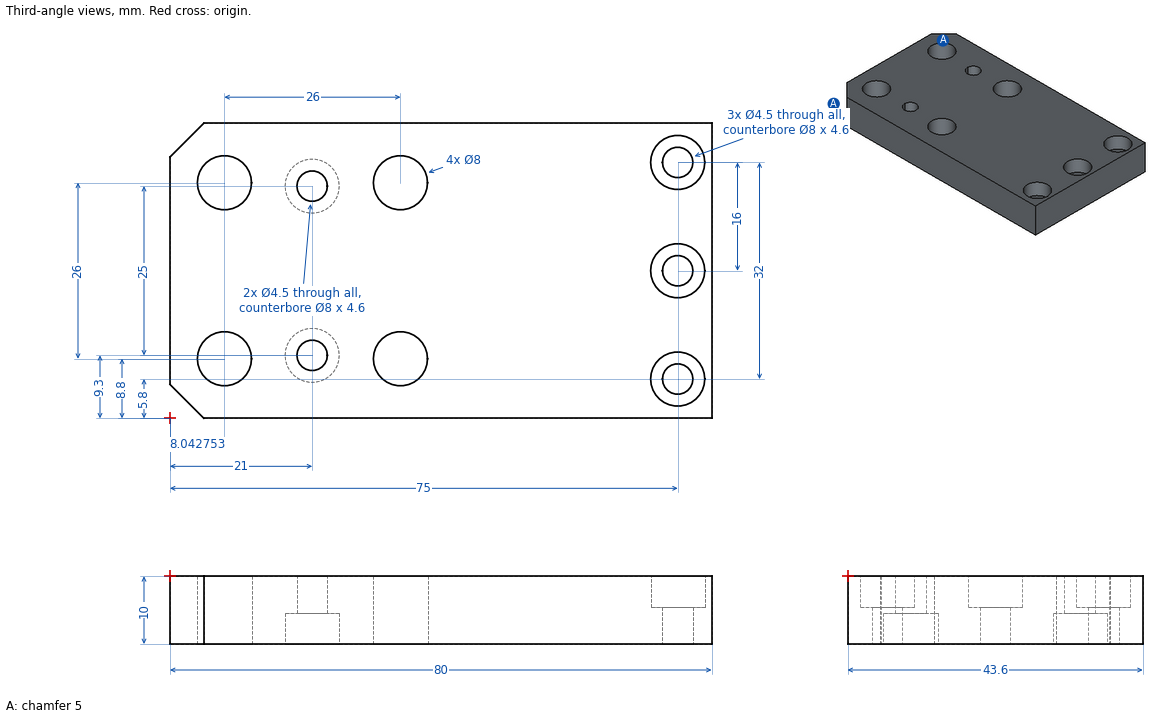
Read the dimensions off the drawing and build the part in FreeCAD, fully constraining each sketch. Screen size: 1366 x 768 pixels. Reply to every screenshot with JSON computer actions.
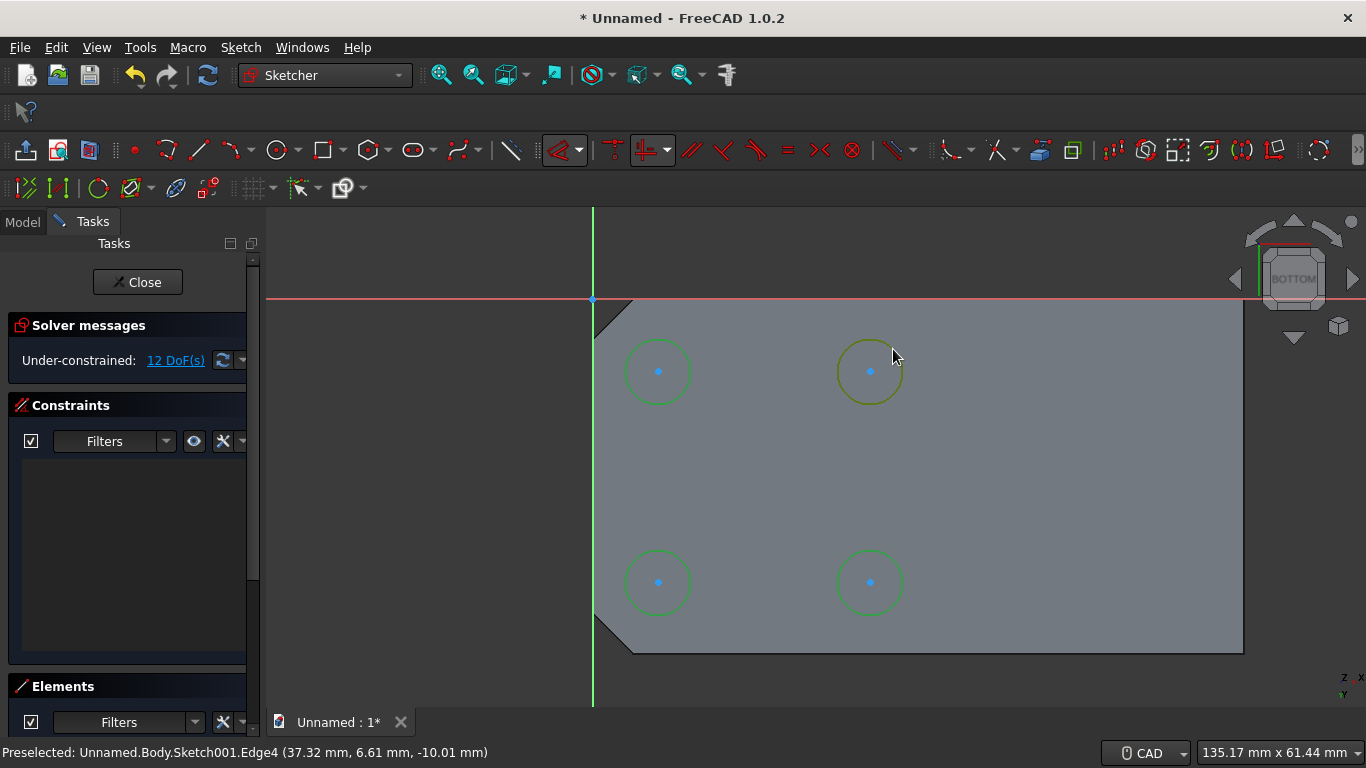
{"action": "left_click", "coordinate": [788, 150]}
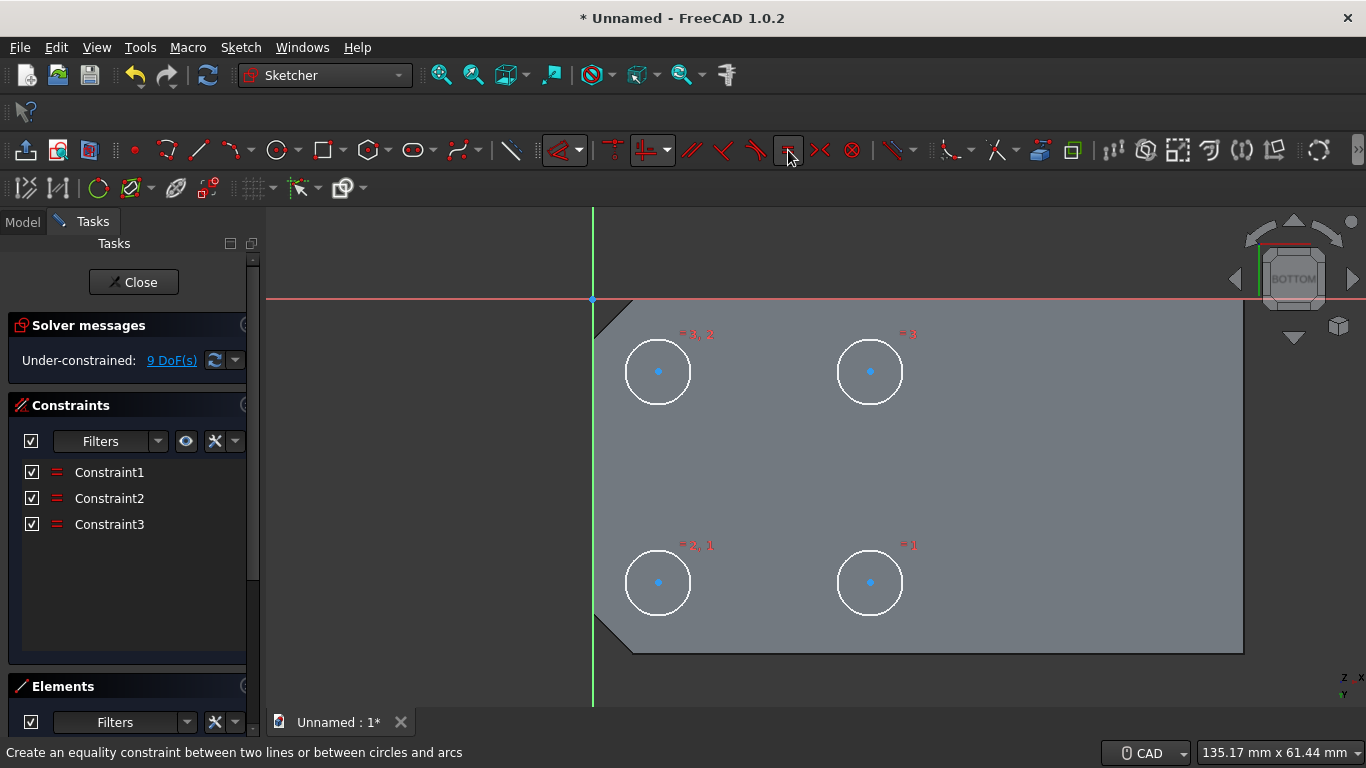
{"action": "left_click", "coordinate": [893, 560]}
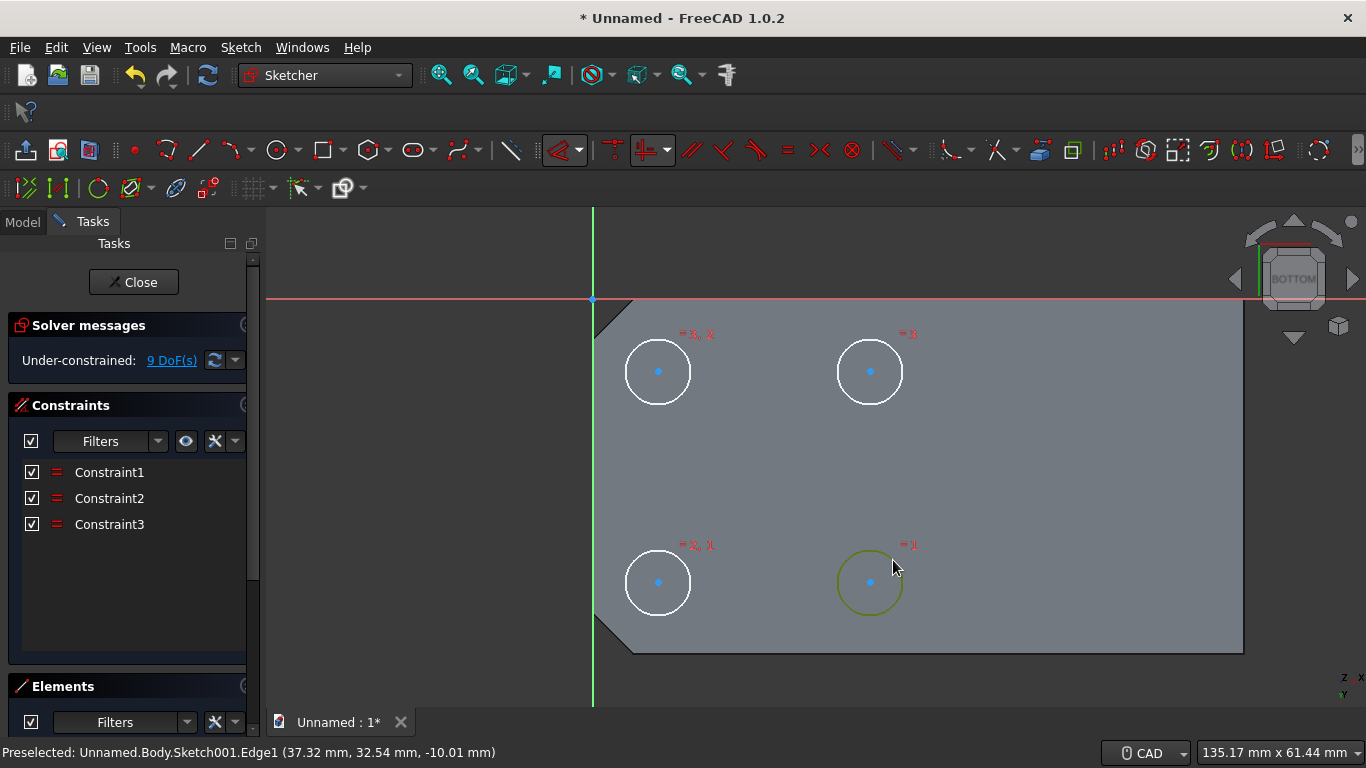
{"action": "left_click", "coordinate": [582, 150]}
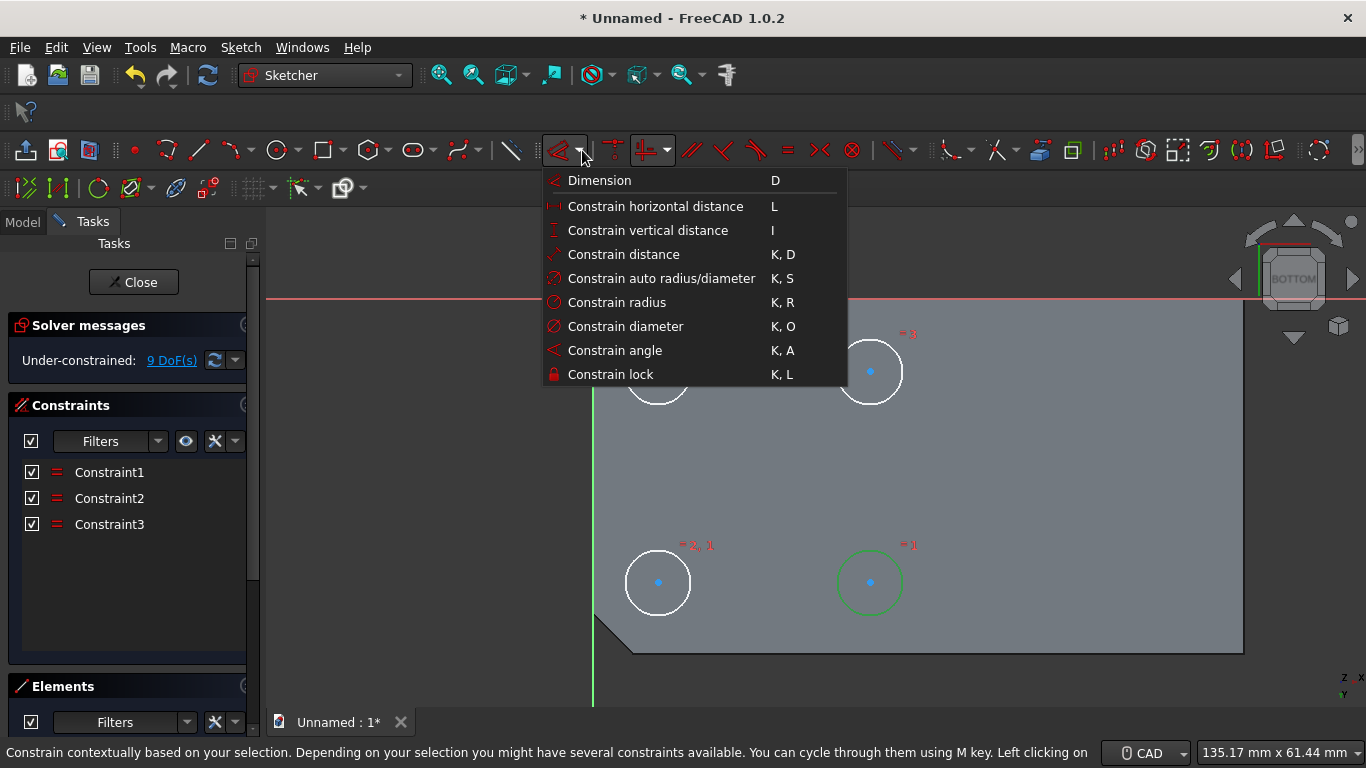
{"action": "left_click", "coordinate": [695, 326]}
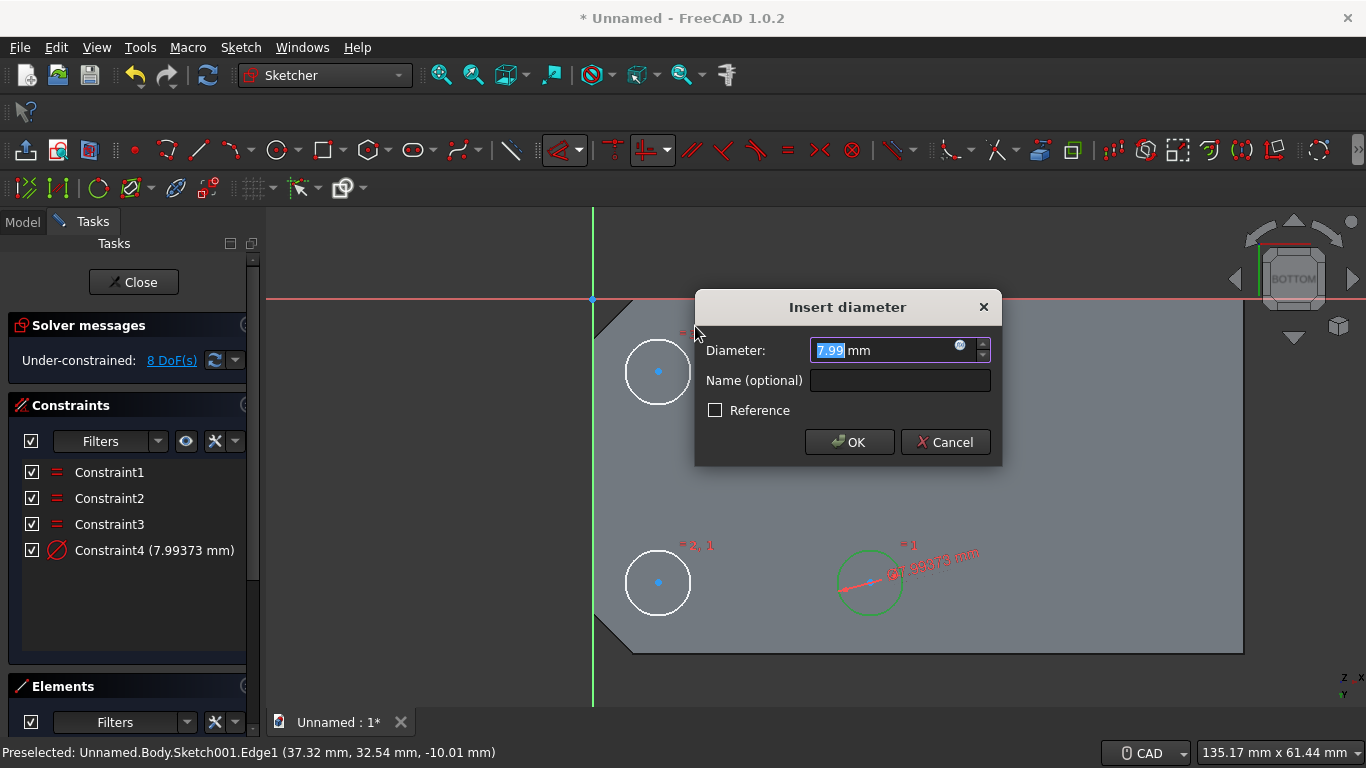
{"action": "type", "text": "8"}
{"action": "key", "text": "Return"}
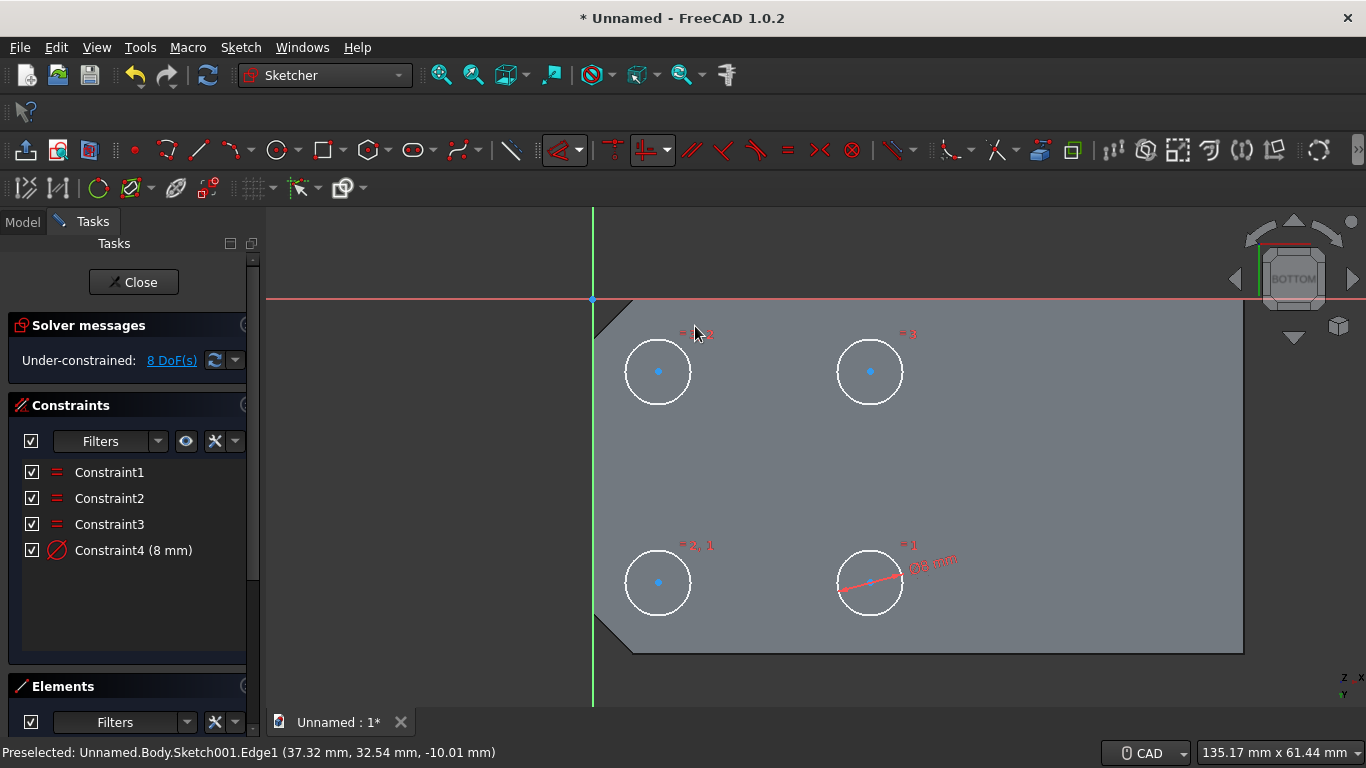
{"action": "left_click", "coordinate": [658, 372]}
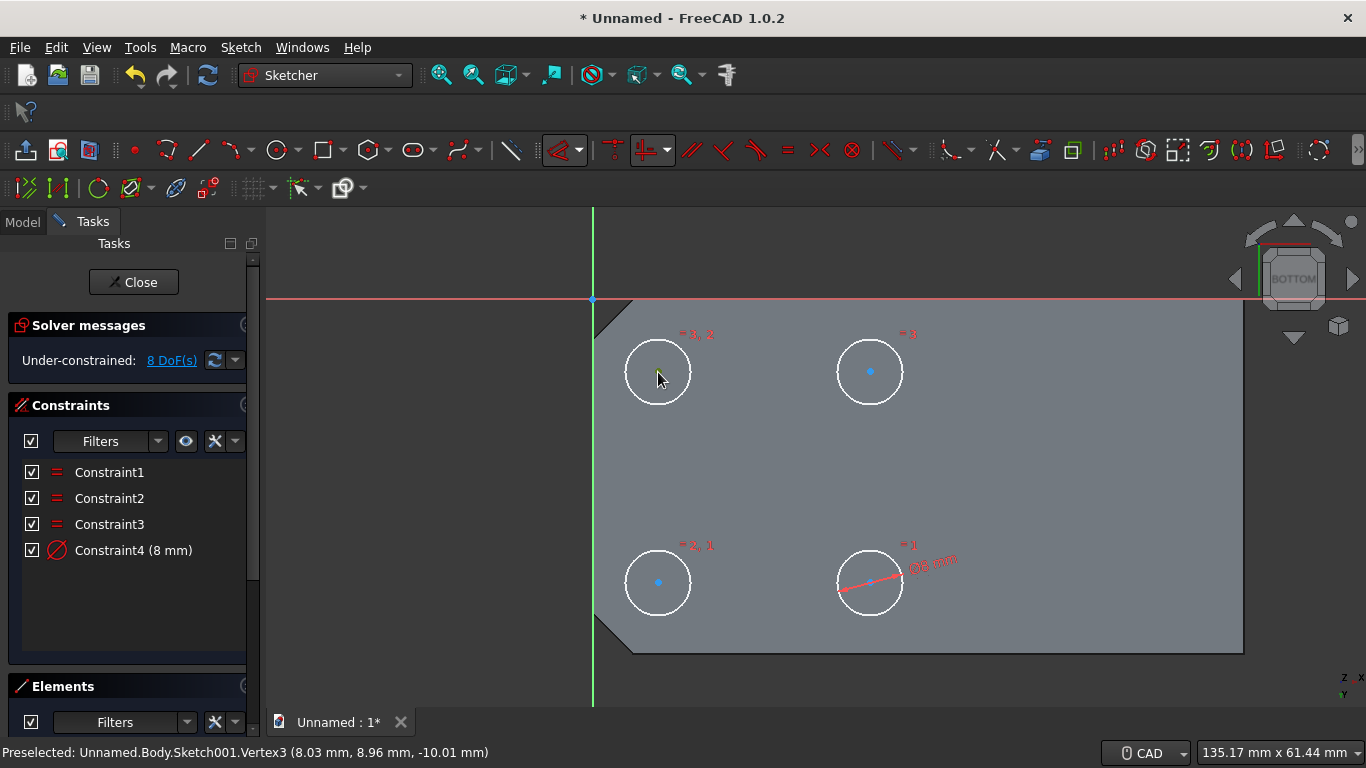
{"action": "left_click", "coordinate": [582, 150]}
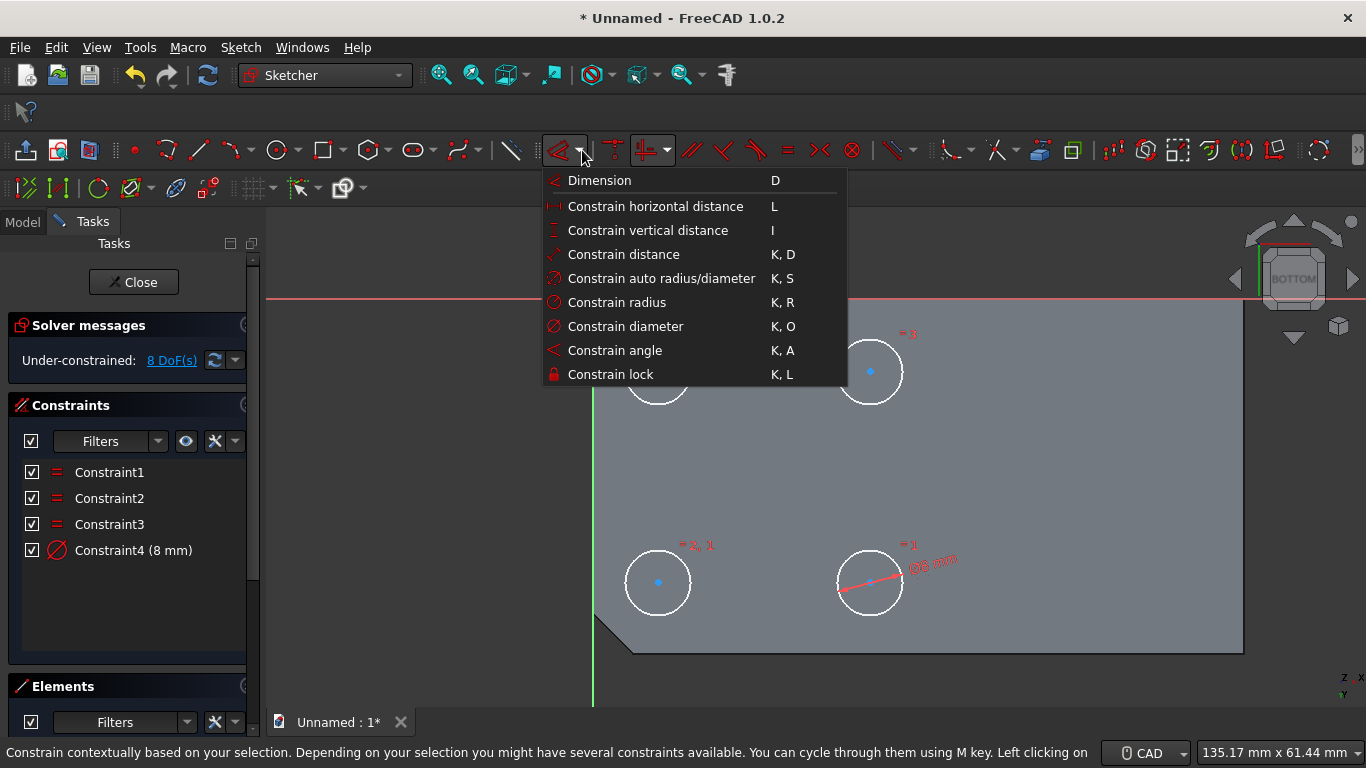
{"action": "left_click", "coordinate": [695, 230]}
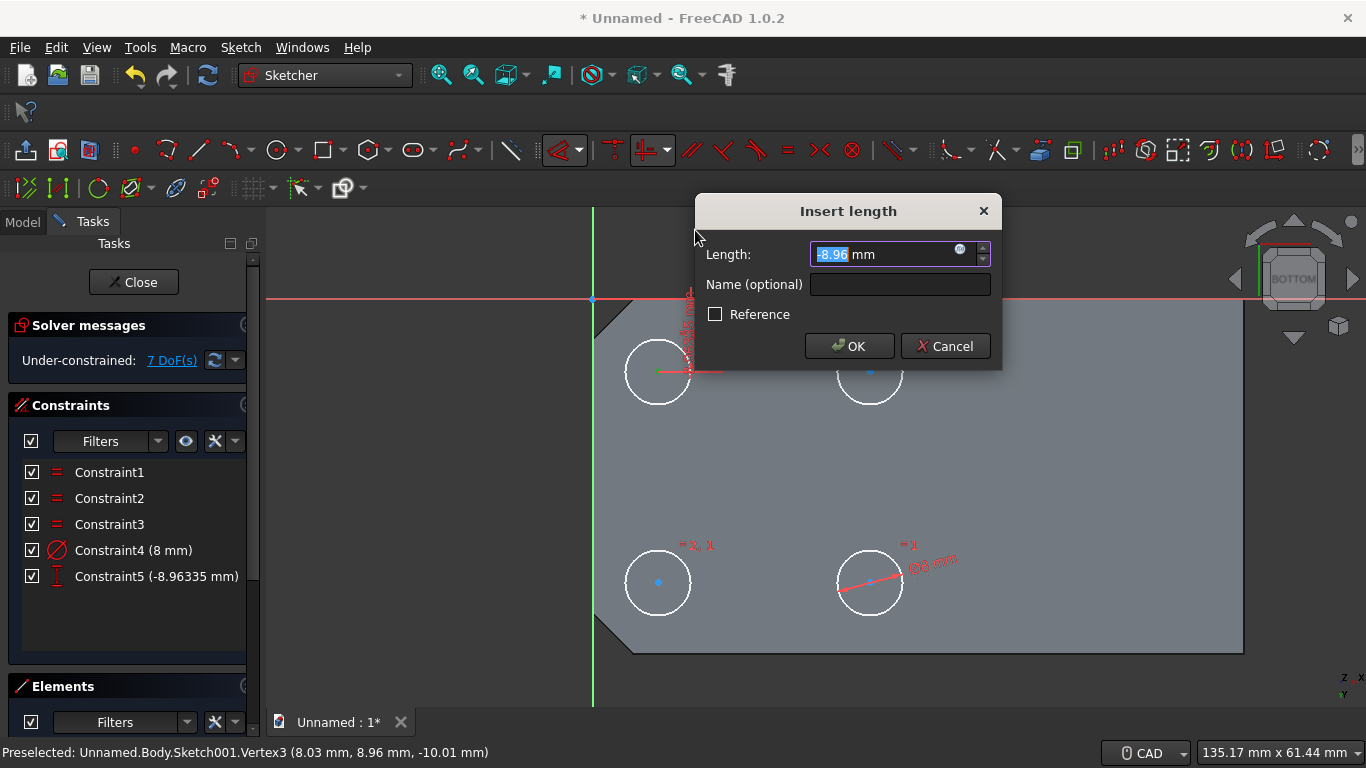
{"action": "type", "text": "-8.8"}
{"action": "key", "text": "Return"}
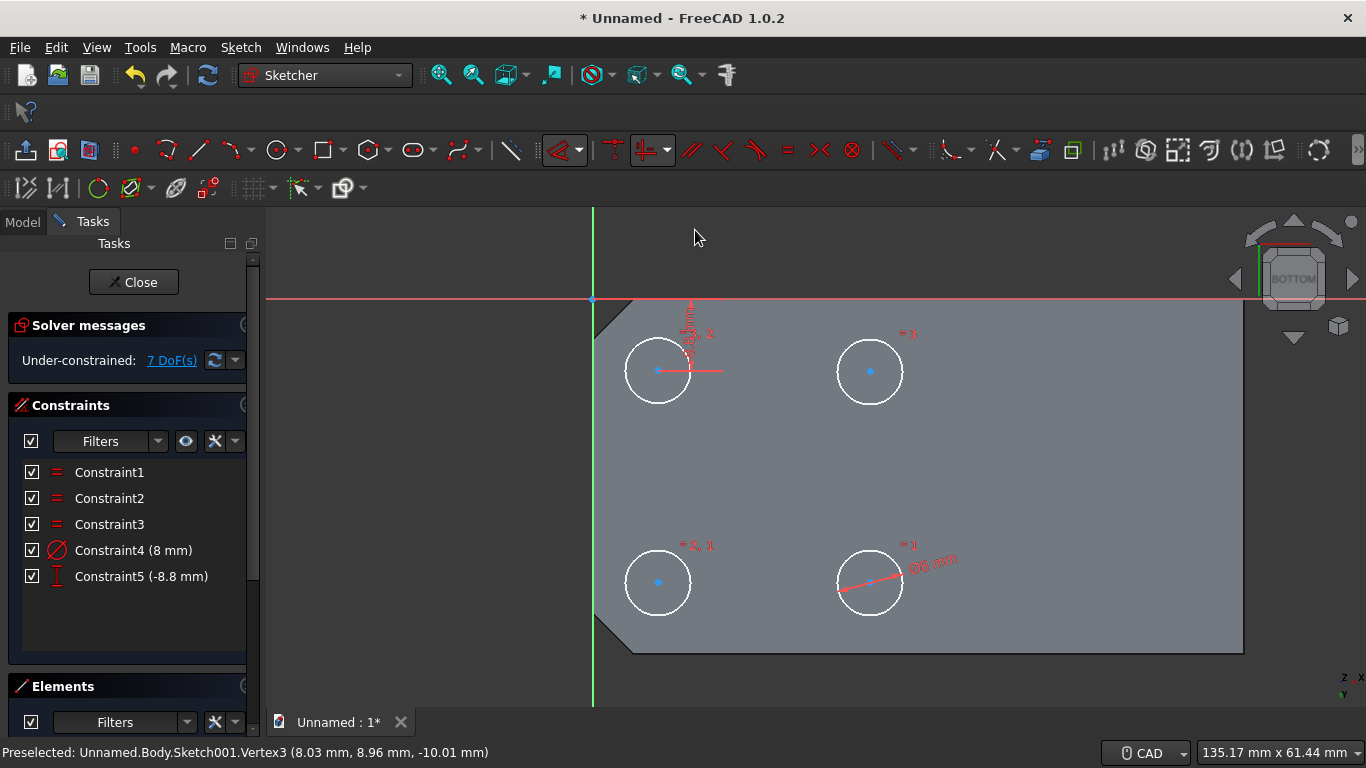
{"action": "left_click", "coordinate": [870, 372]}